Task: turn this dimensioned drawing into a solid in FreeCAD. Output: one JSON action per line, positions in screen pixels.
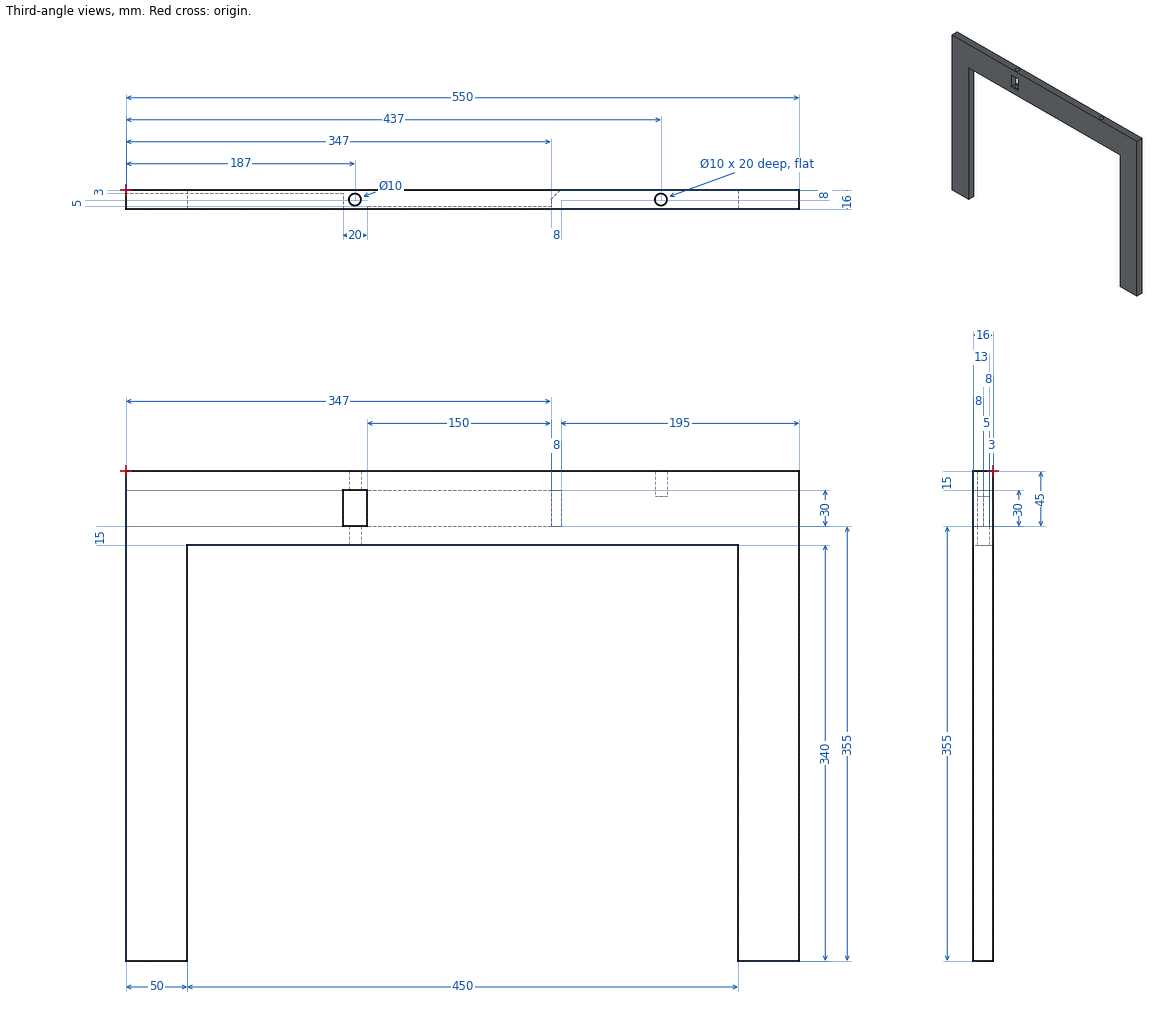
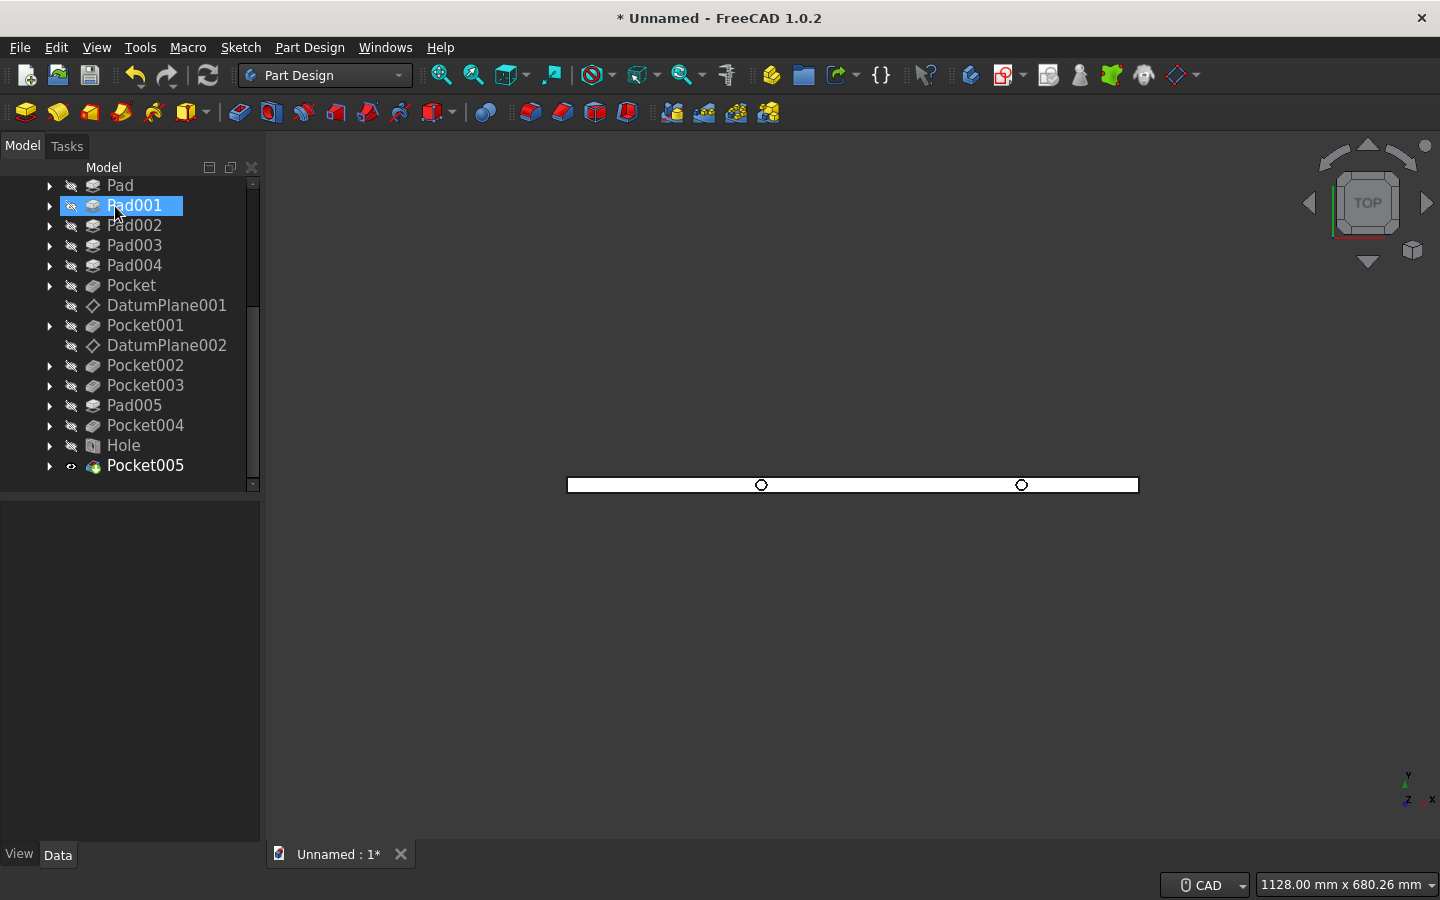
{"action": "scroll", "coordinate": [140, 321], "scroll_direction": "down", "scroll_amount": 3}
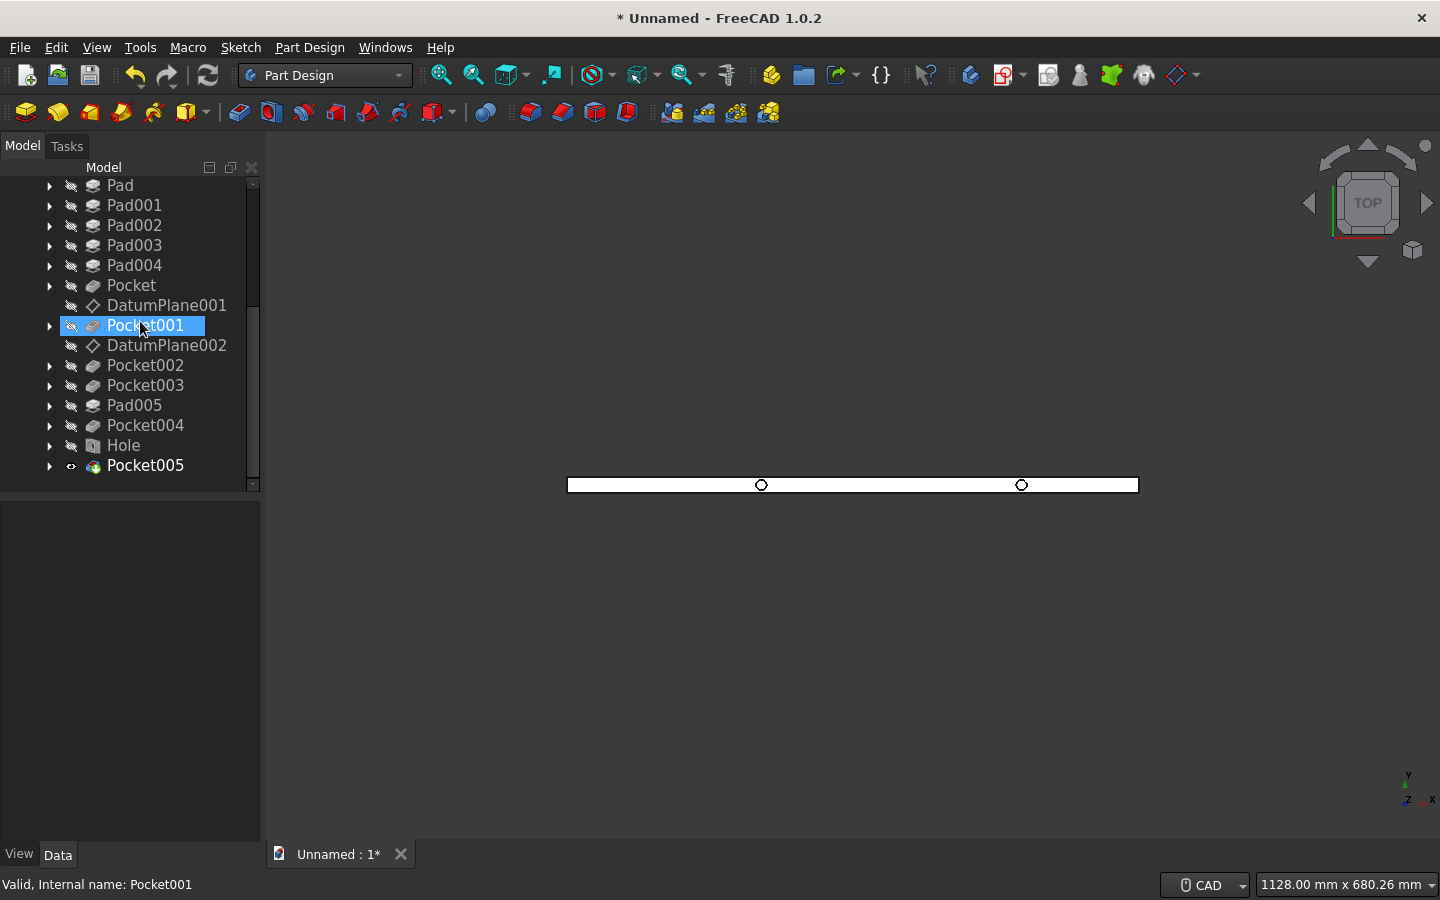
{"action": "scroll", "coordinate": [140, 321], "scroll_direction": "up", "scroll_amount": 15}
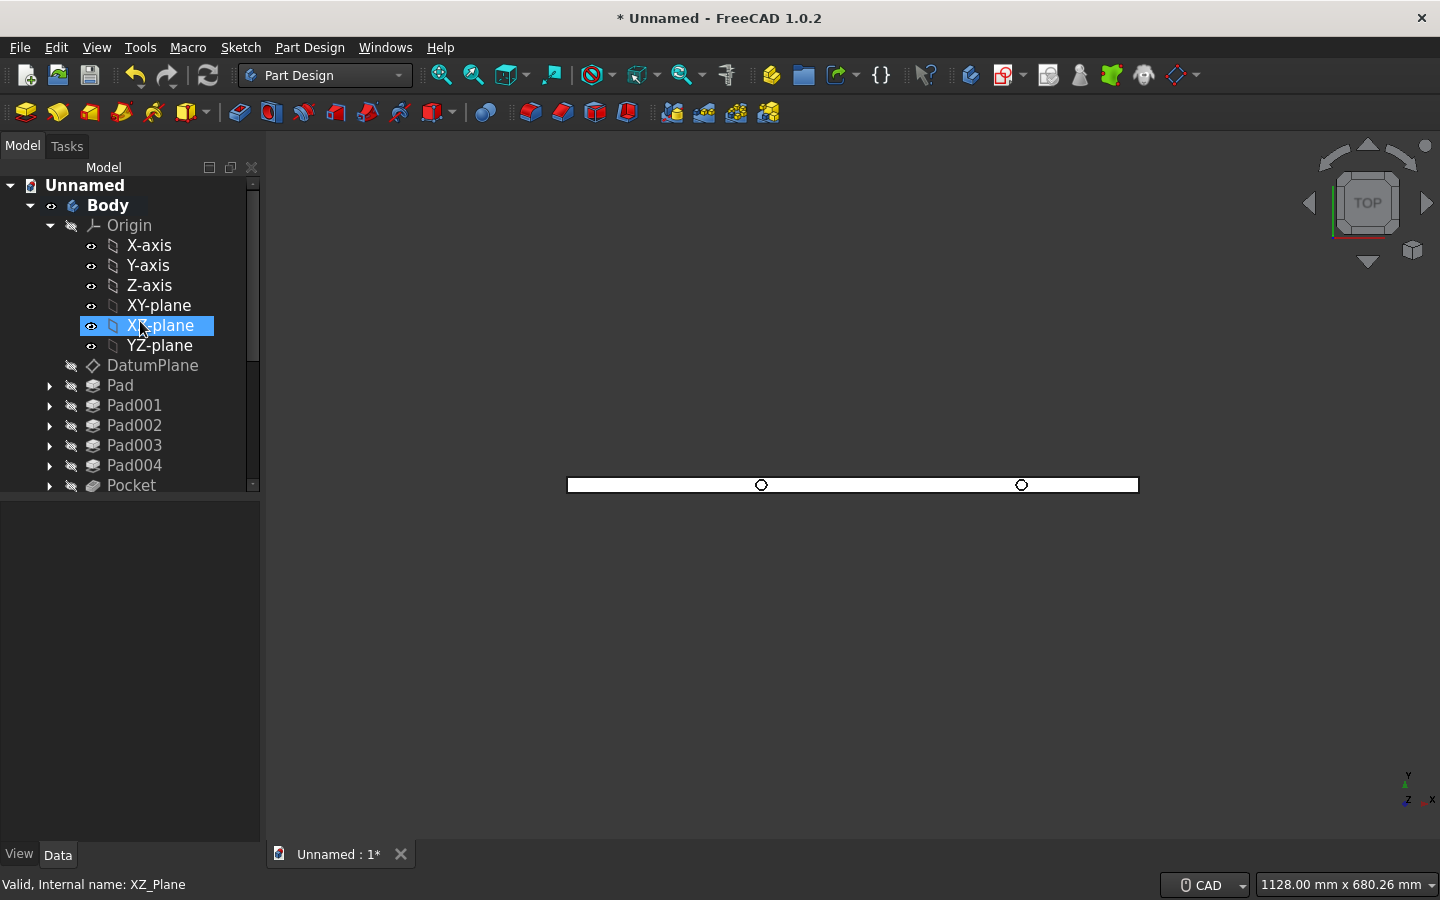
{"action": "left_click", "coordinate": [136, 306]}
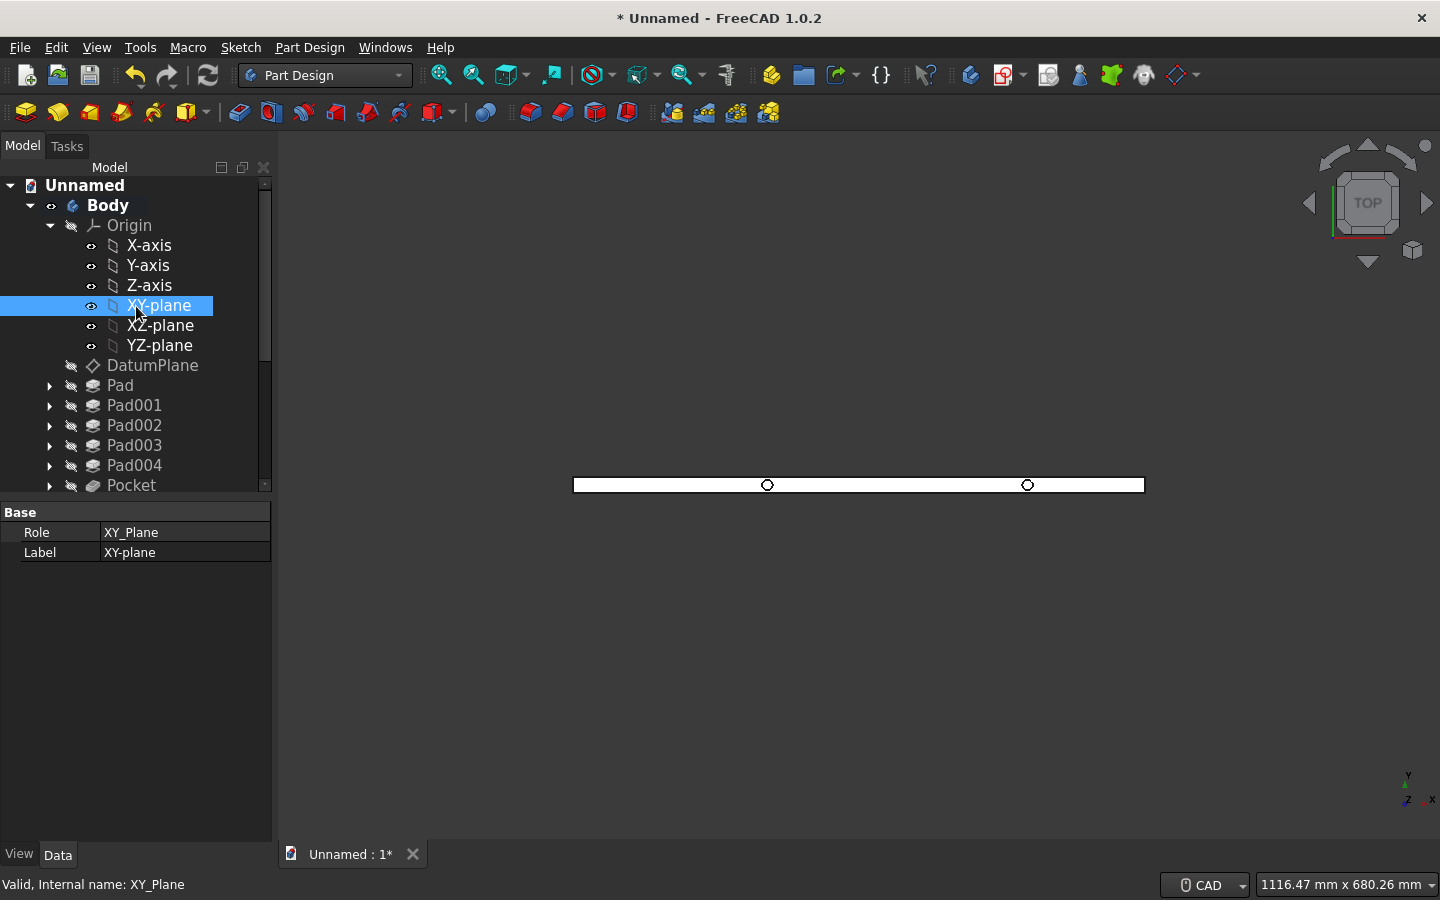
{"action": "left_click", "coordinate": [1176, 76]}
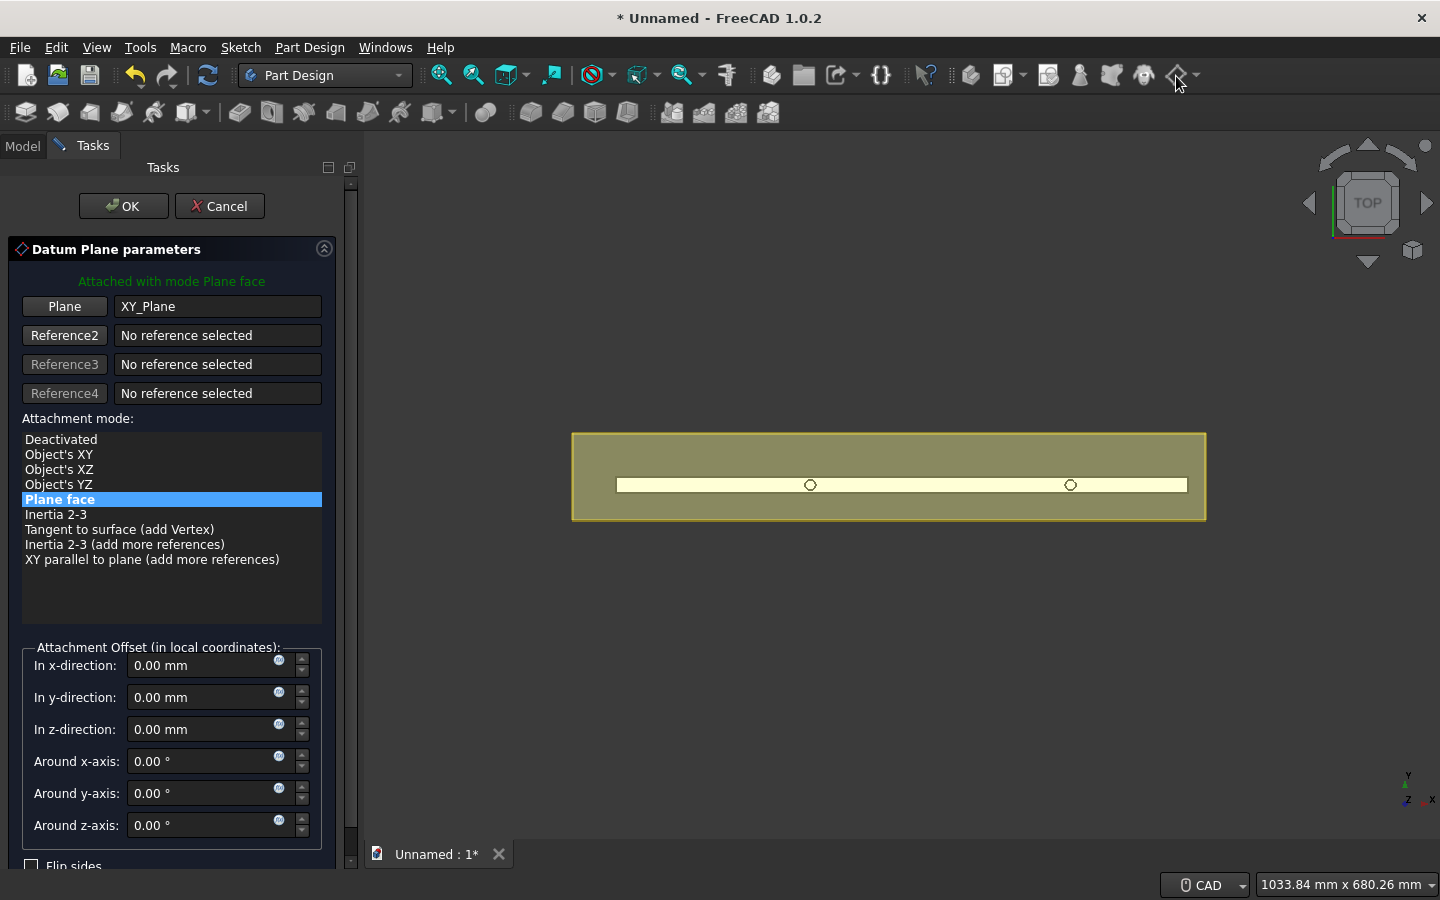
{"action": "triple_click", "coordinate": [210, 729]}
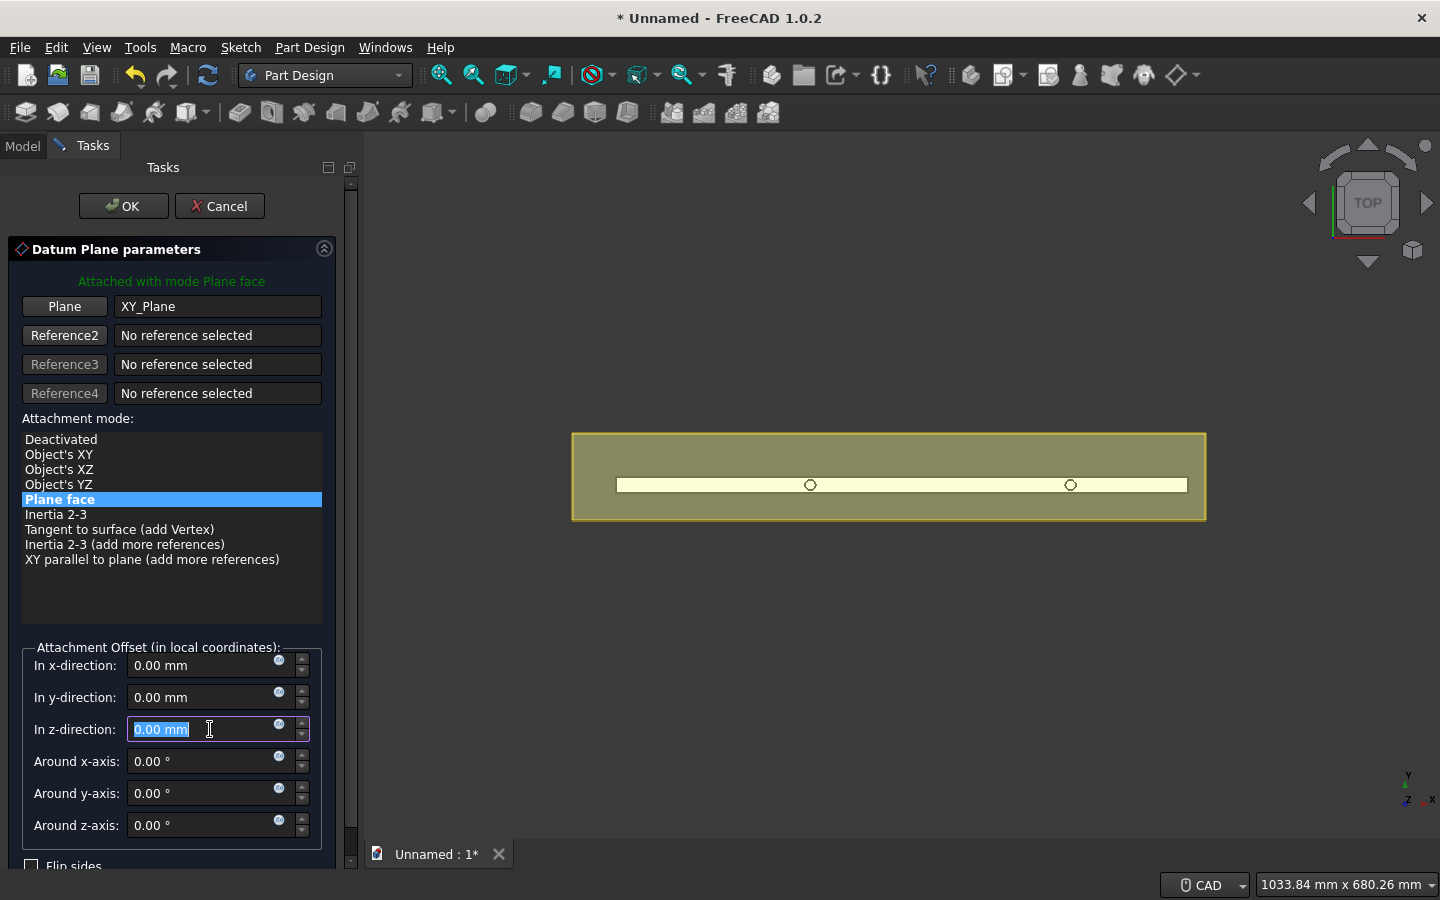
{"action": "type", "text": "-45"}
{"action": "key", "text": "Tab"}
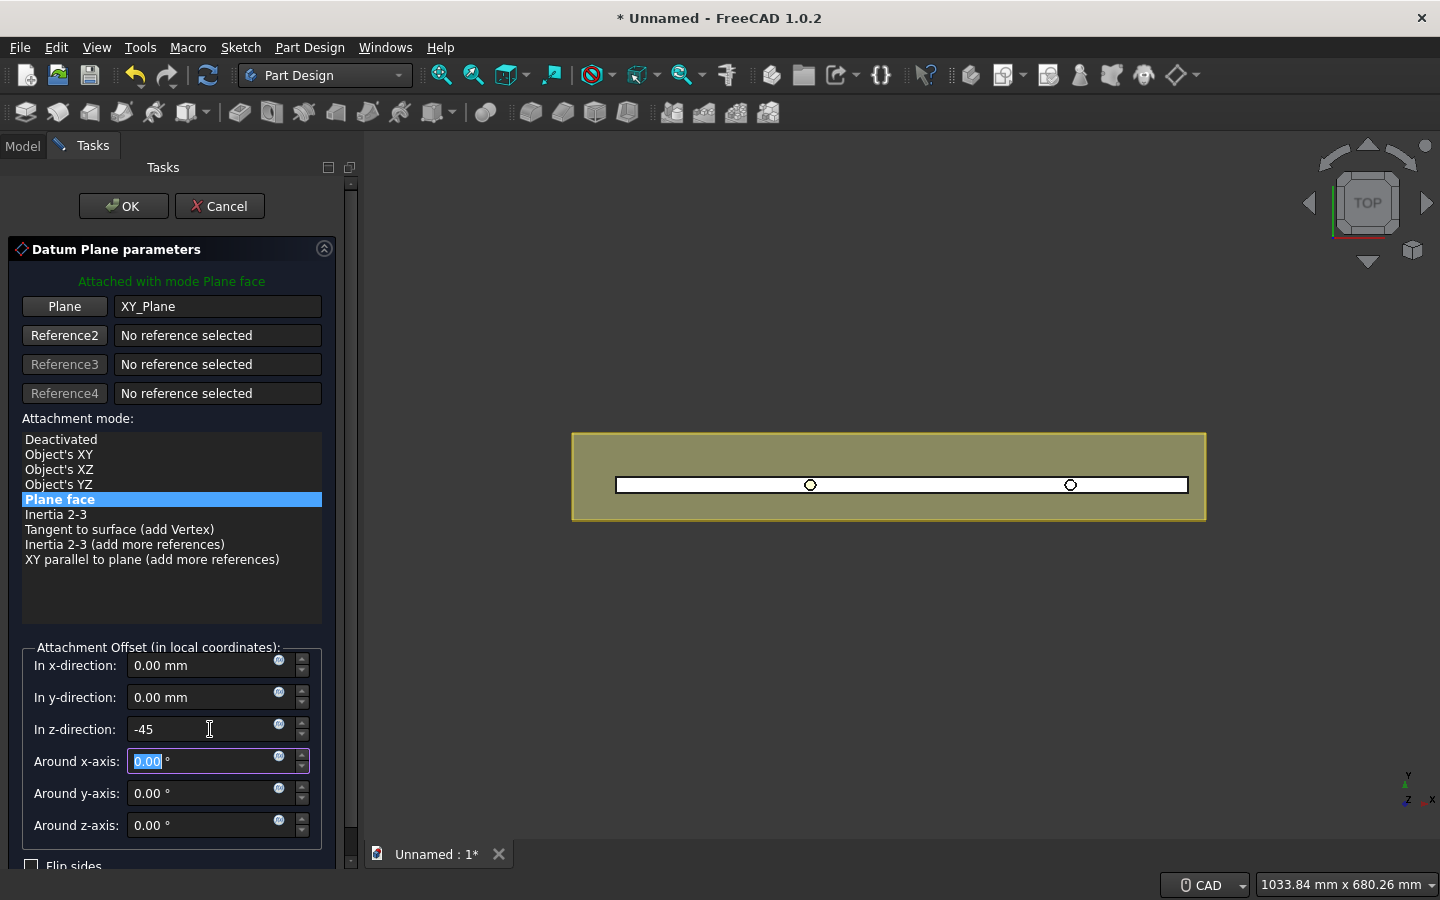
{"action": "left_click", "coordinate": [124, 206]}